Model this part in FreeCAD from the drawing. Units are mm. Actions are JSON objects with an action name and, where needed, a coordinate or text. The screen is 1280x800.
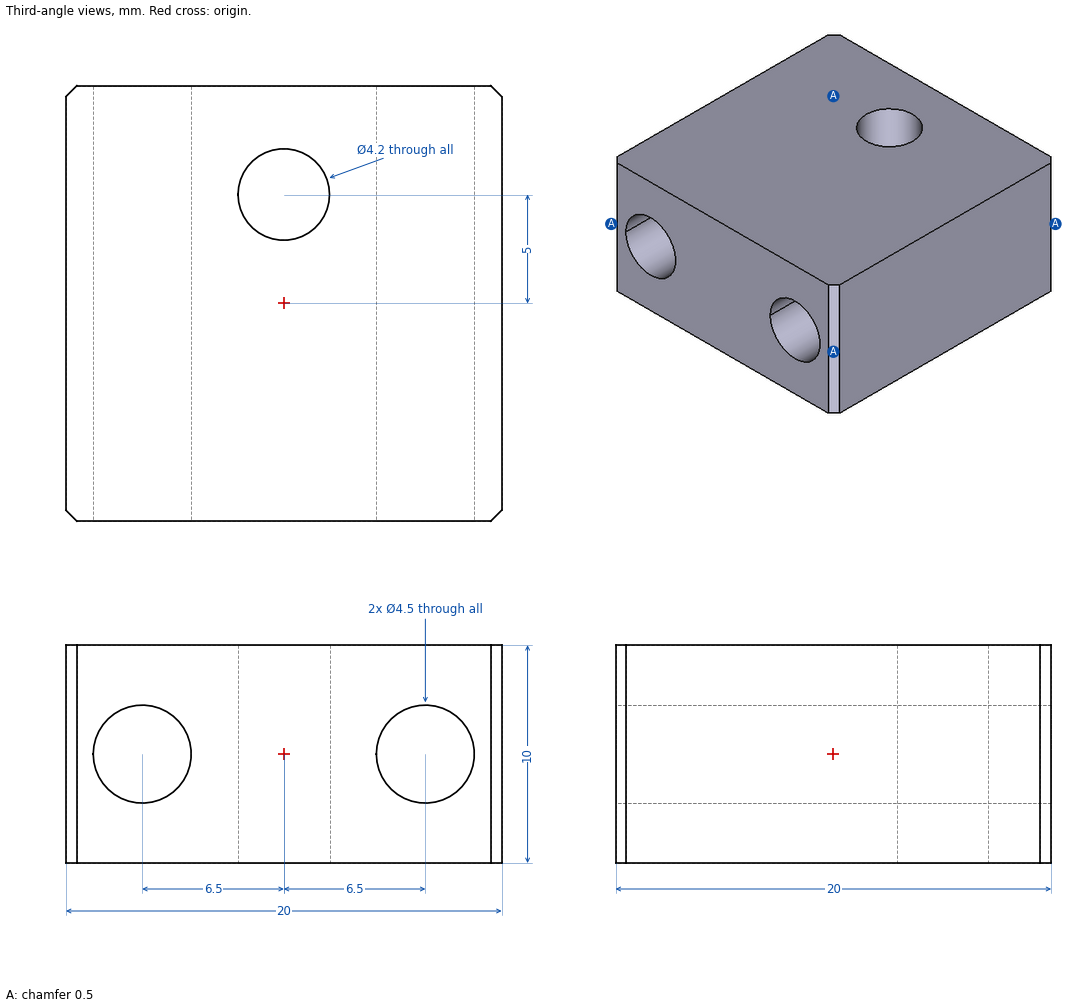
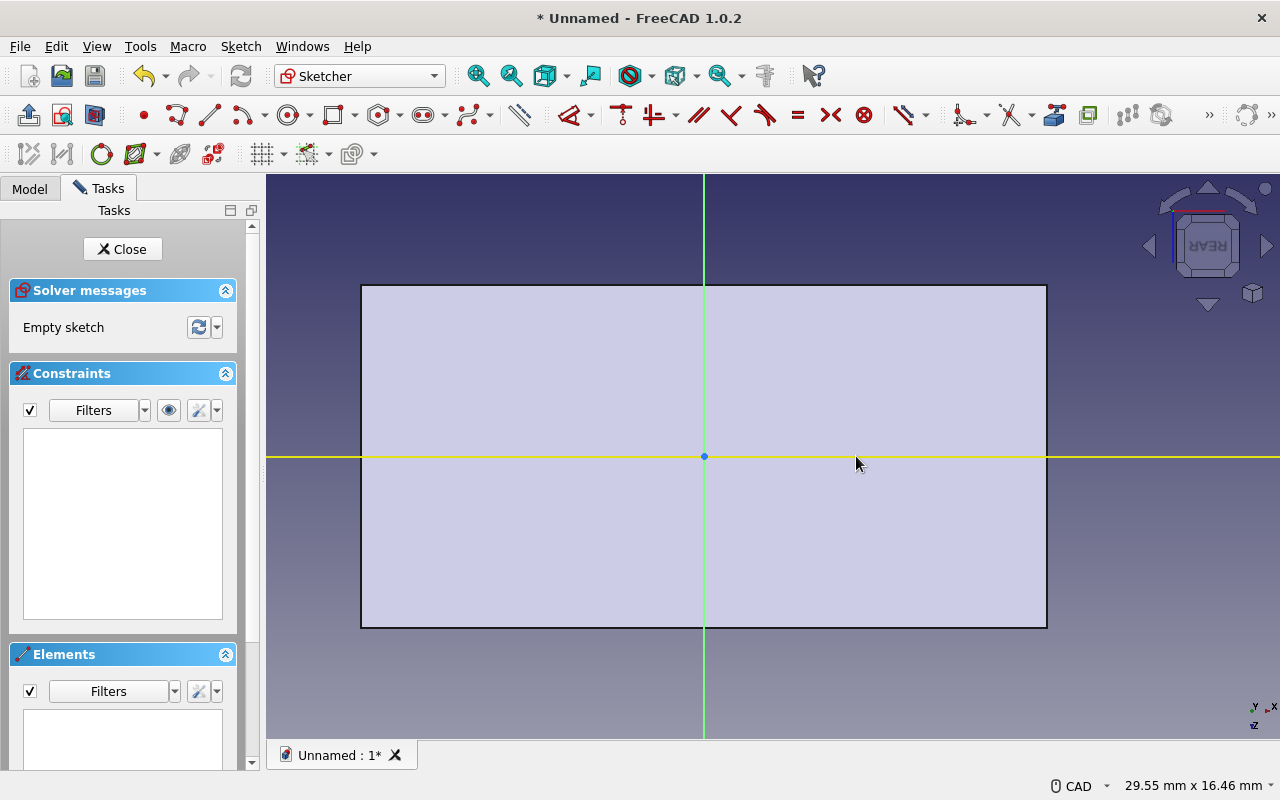
{"action": "left_click", "coordinate": [288, 116]}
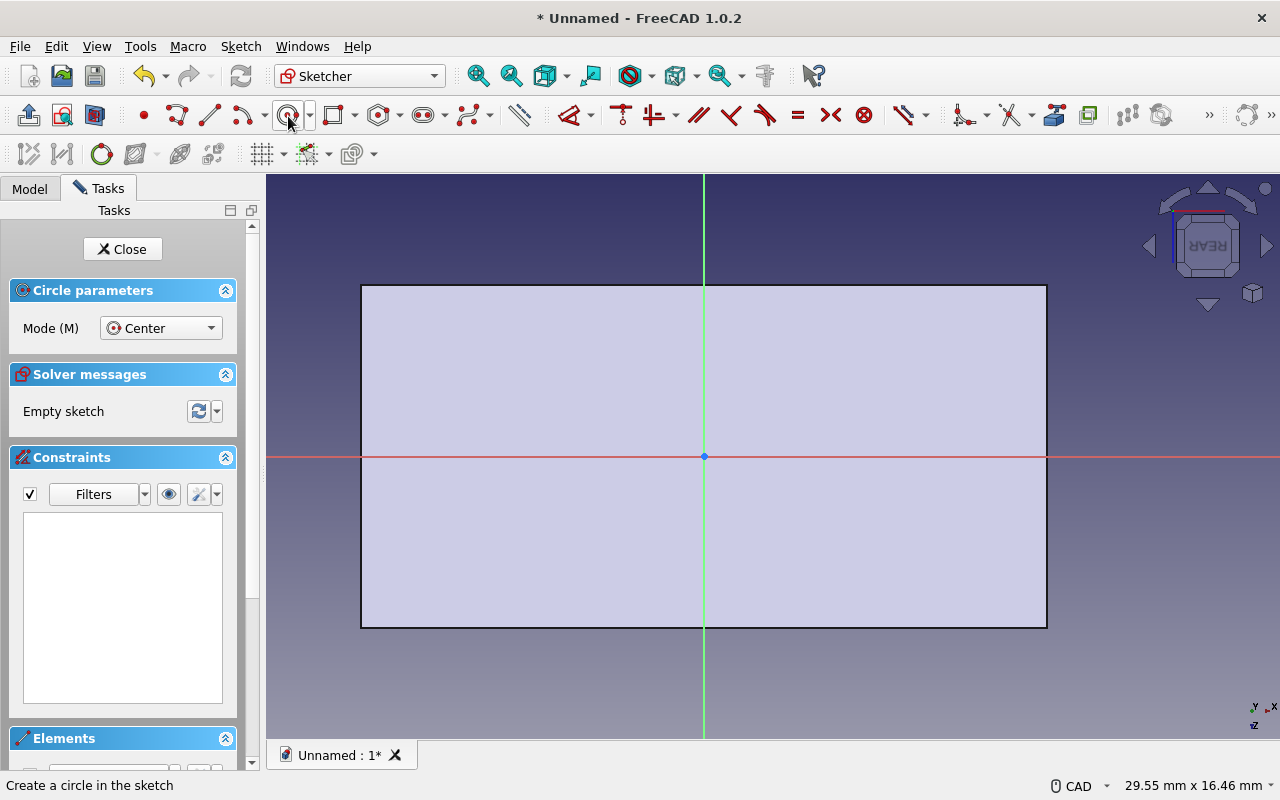
{"action": "left_click", "coordinate": [927, 456]}
{"action": "left_click", "coordinate": [982, 402]}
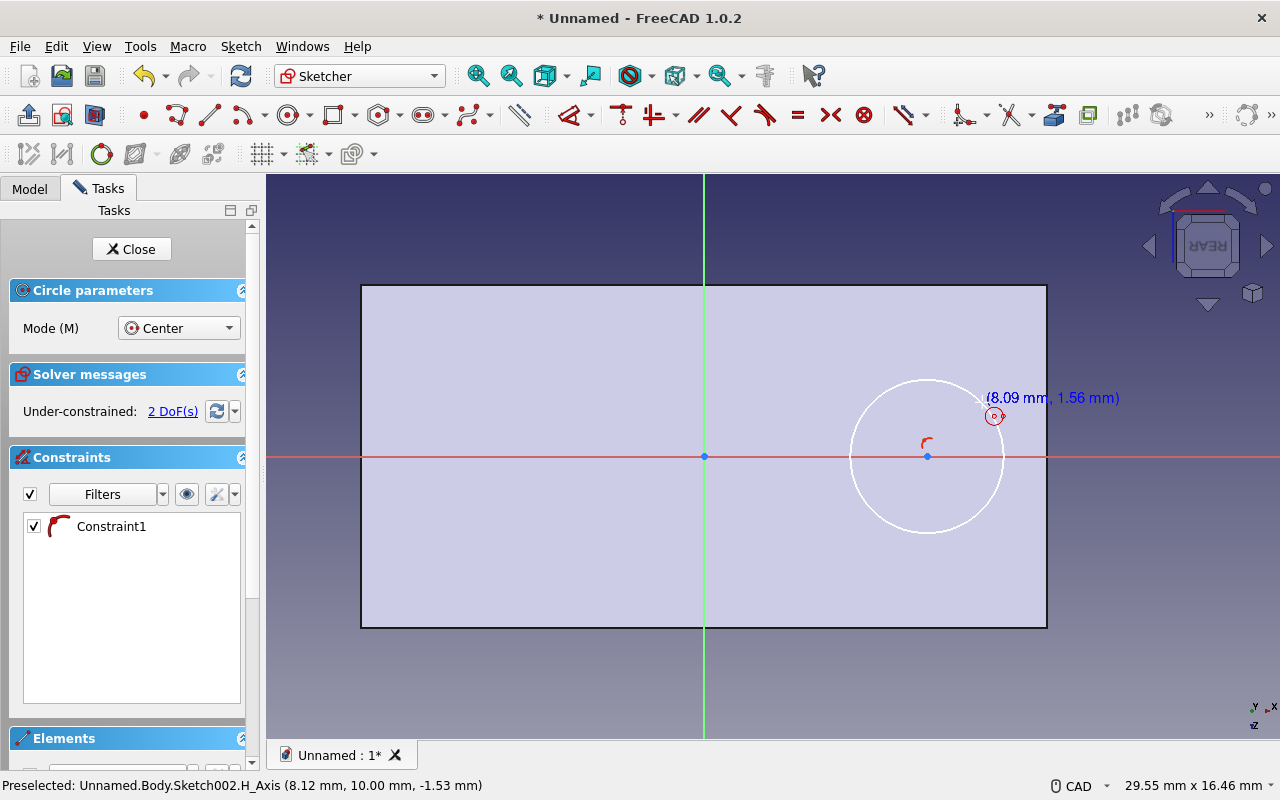
{"action": "left_click", "coordinate": [481, 456]}
{"action": "left_click", "coordinate": [536, 402]}
{"action": "key", "text": "Escape"}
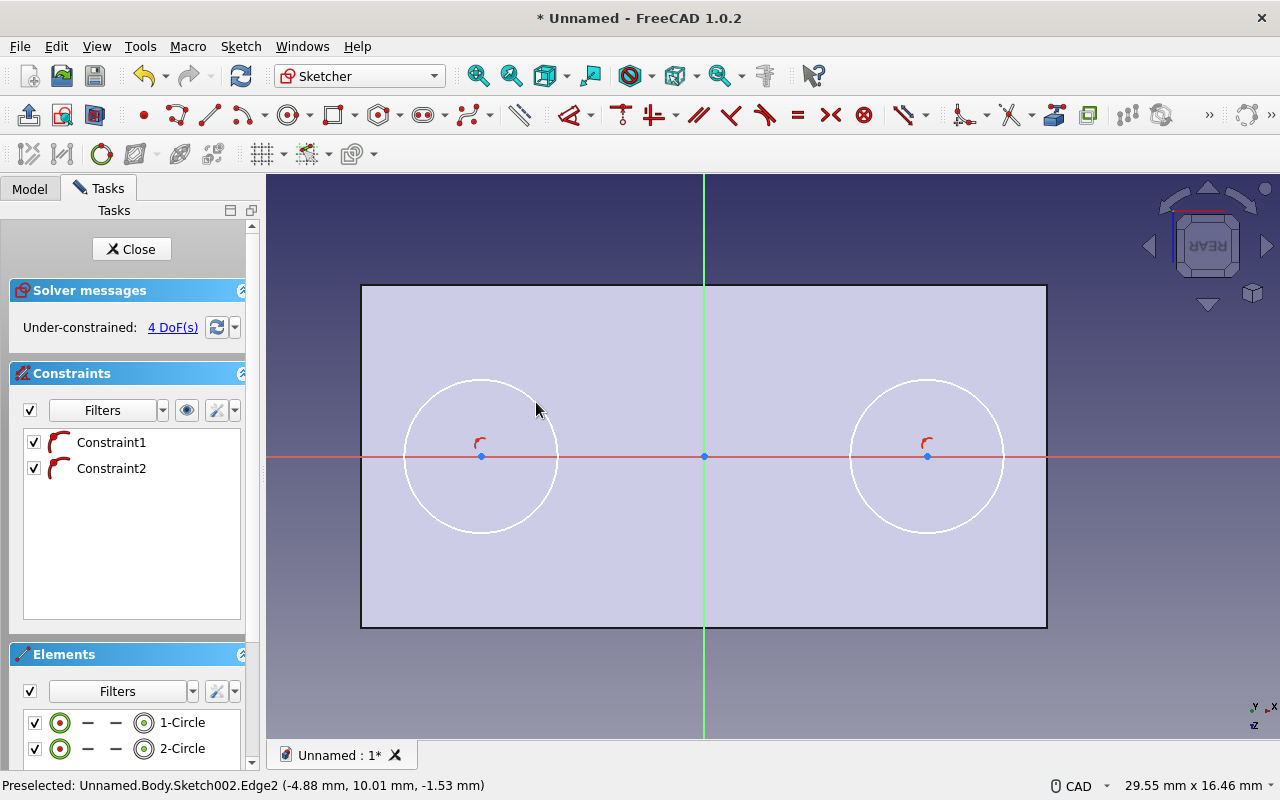
{"action": "left_click", "coordinate": [981, 402]}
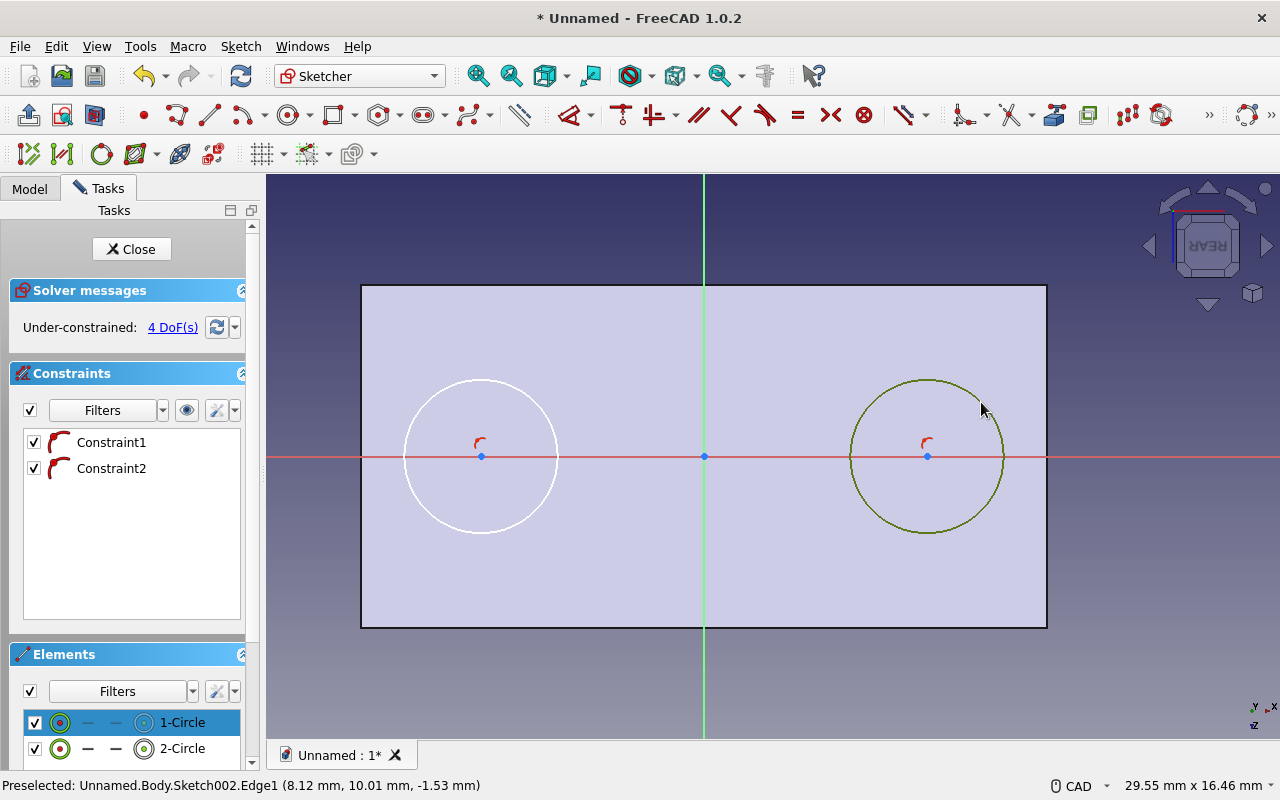
{"action": "left_click", "coordinate": [535, 402]}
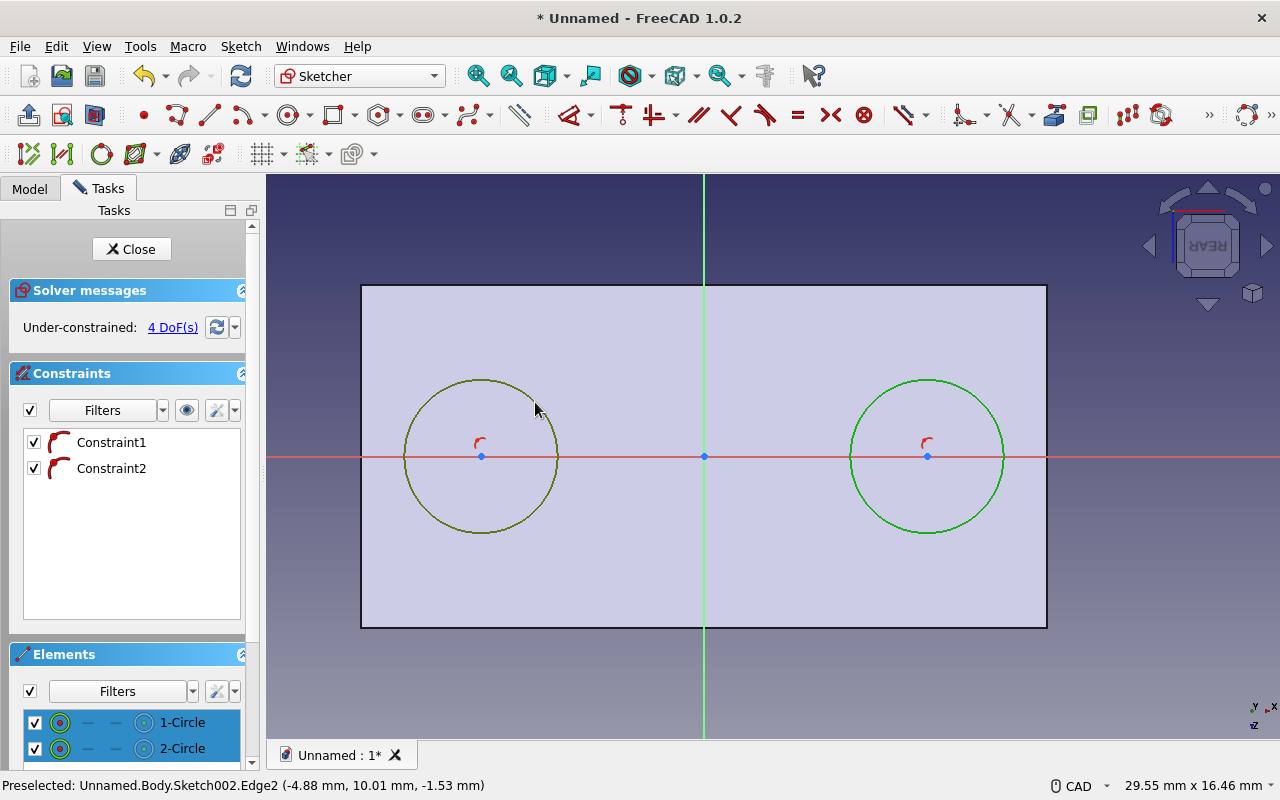
{"action": "key", "text": "e"}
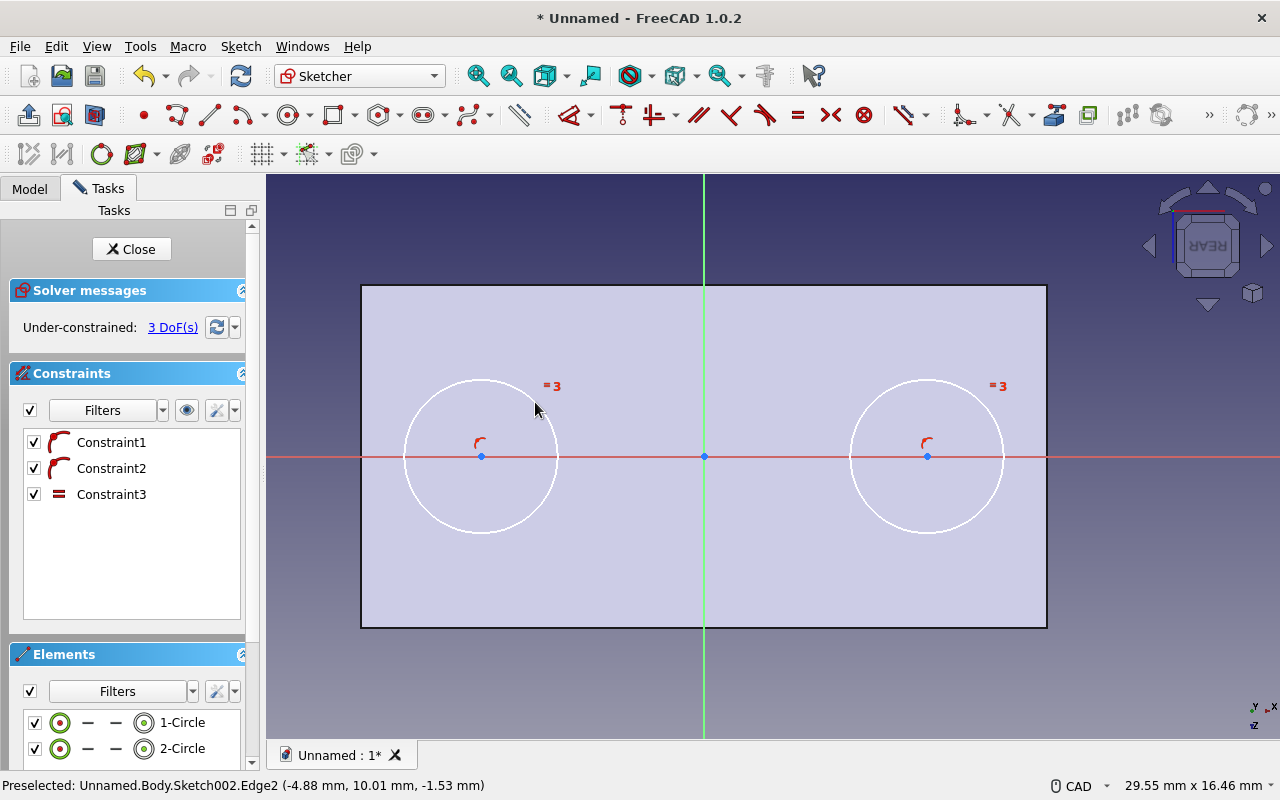
{"action": "key", "text": "d"}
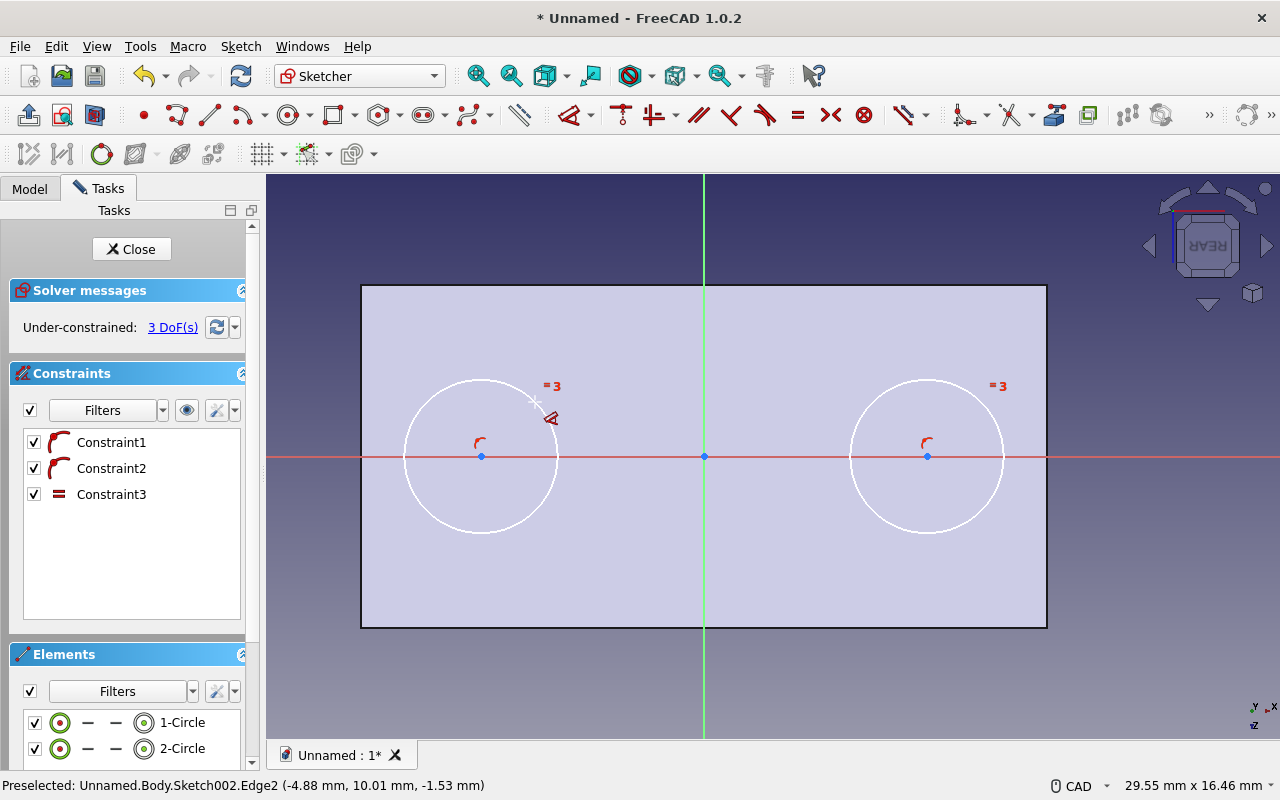
{"action": "left_click", "coordinate": [981, 402]}
{"action": "left_click", "coordinate": [1004, 379]}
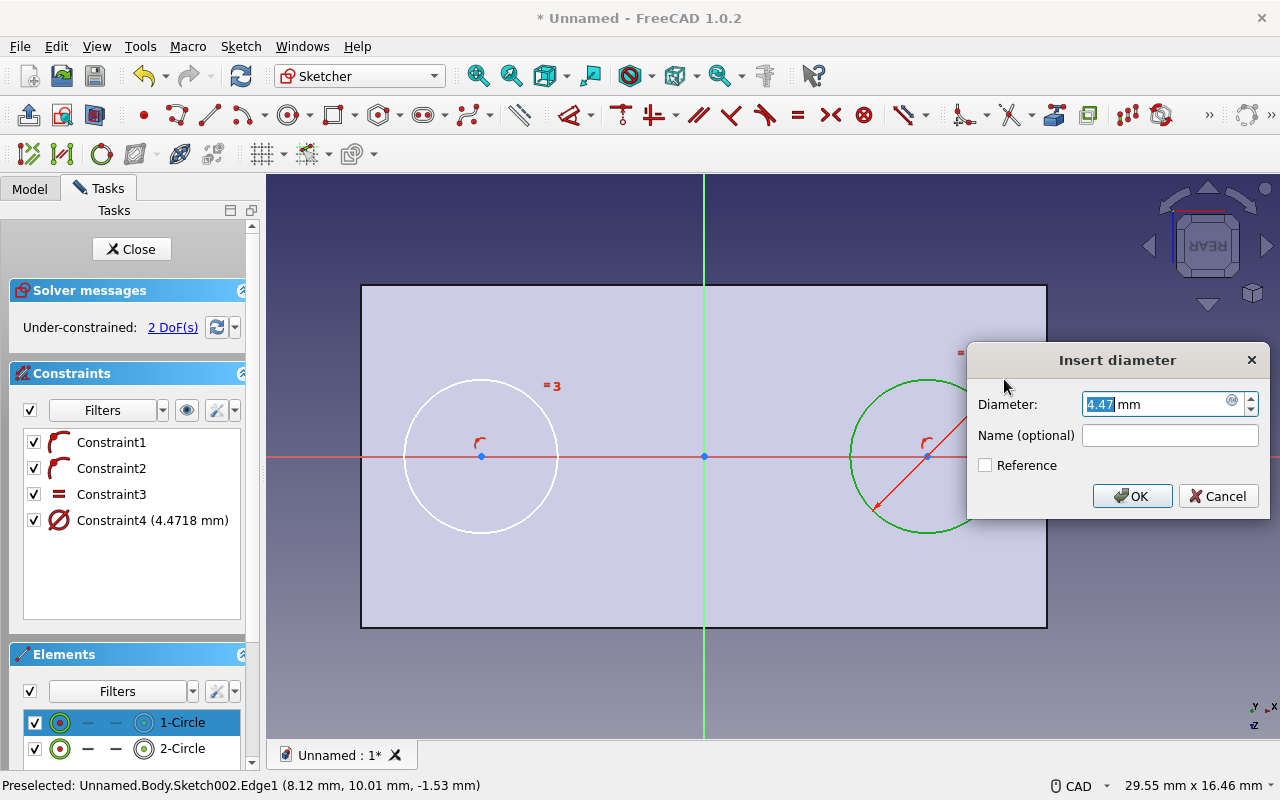
{"action": "type", "text": "4.5"}
{"action": "key", "text": "Return"}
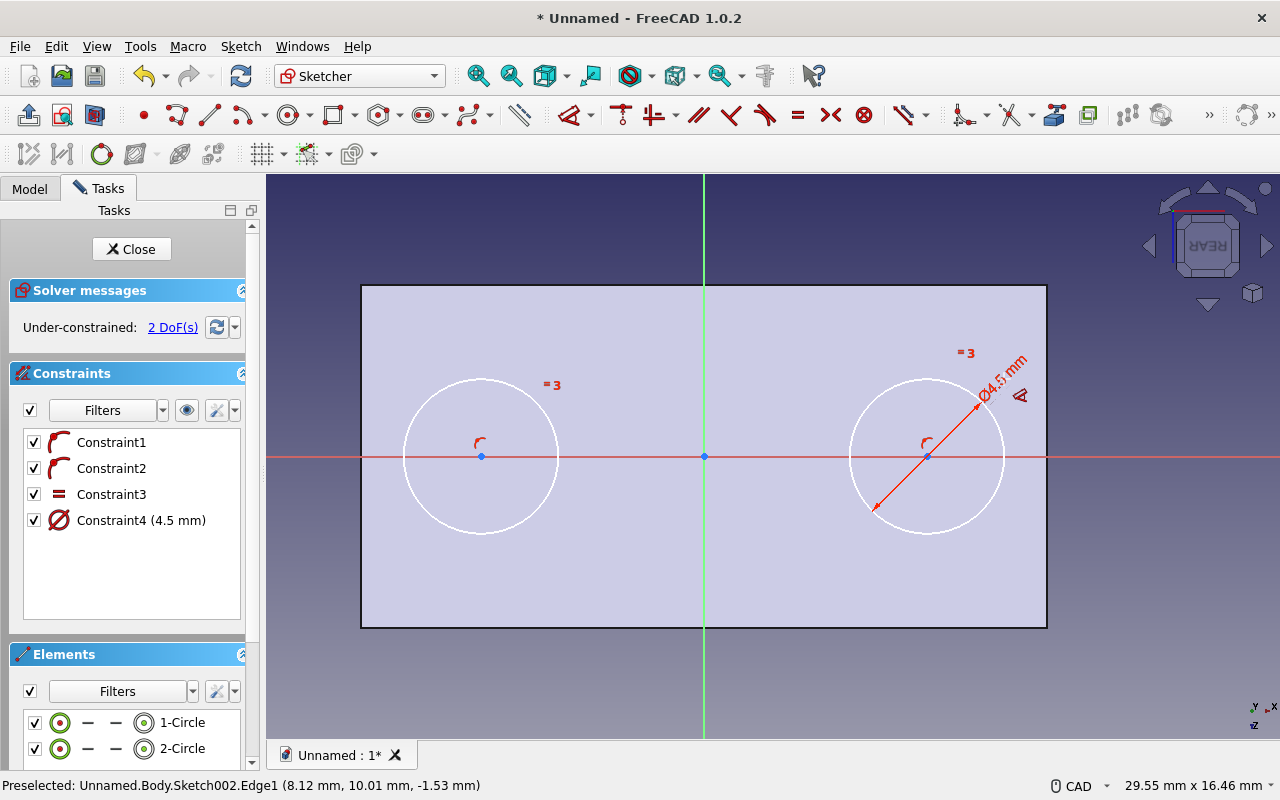
{"action": "left_click", "coordinate": [927, 456]}
{"action": "left_click", "coordinate": [816, 490]}